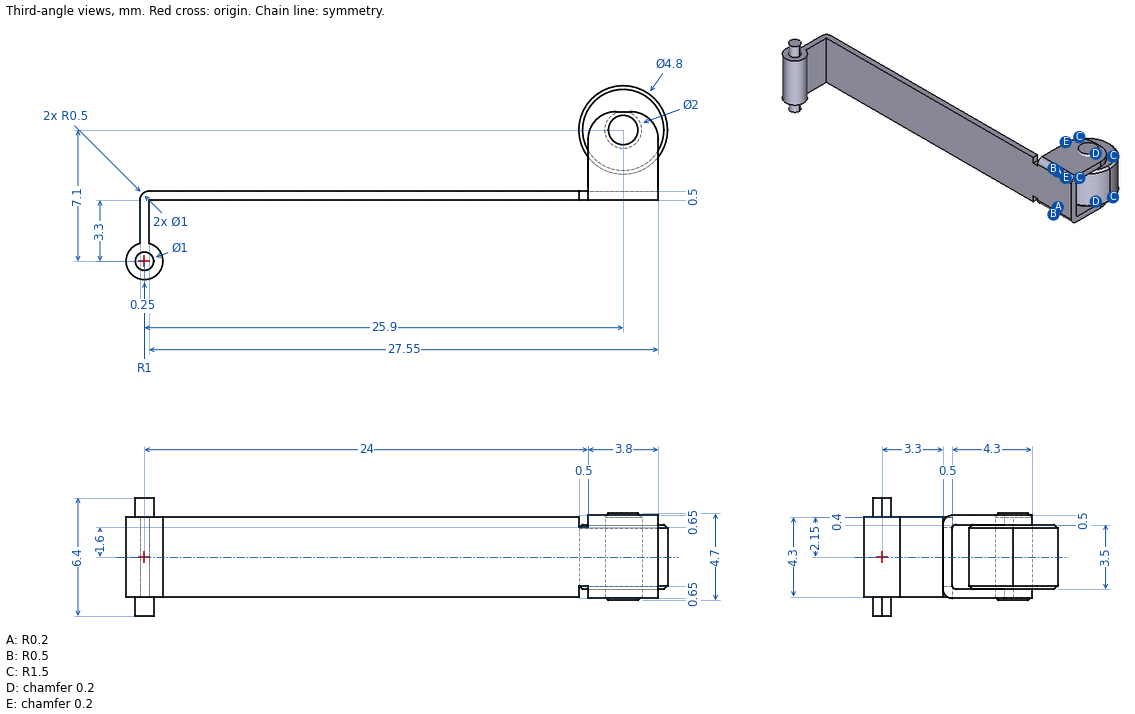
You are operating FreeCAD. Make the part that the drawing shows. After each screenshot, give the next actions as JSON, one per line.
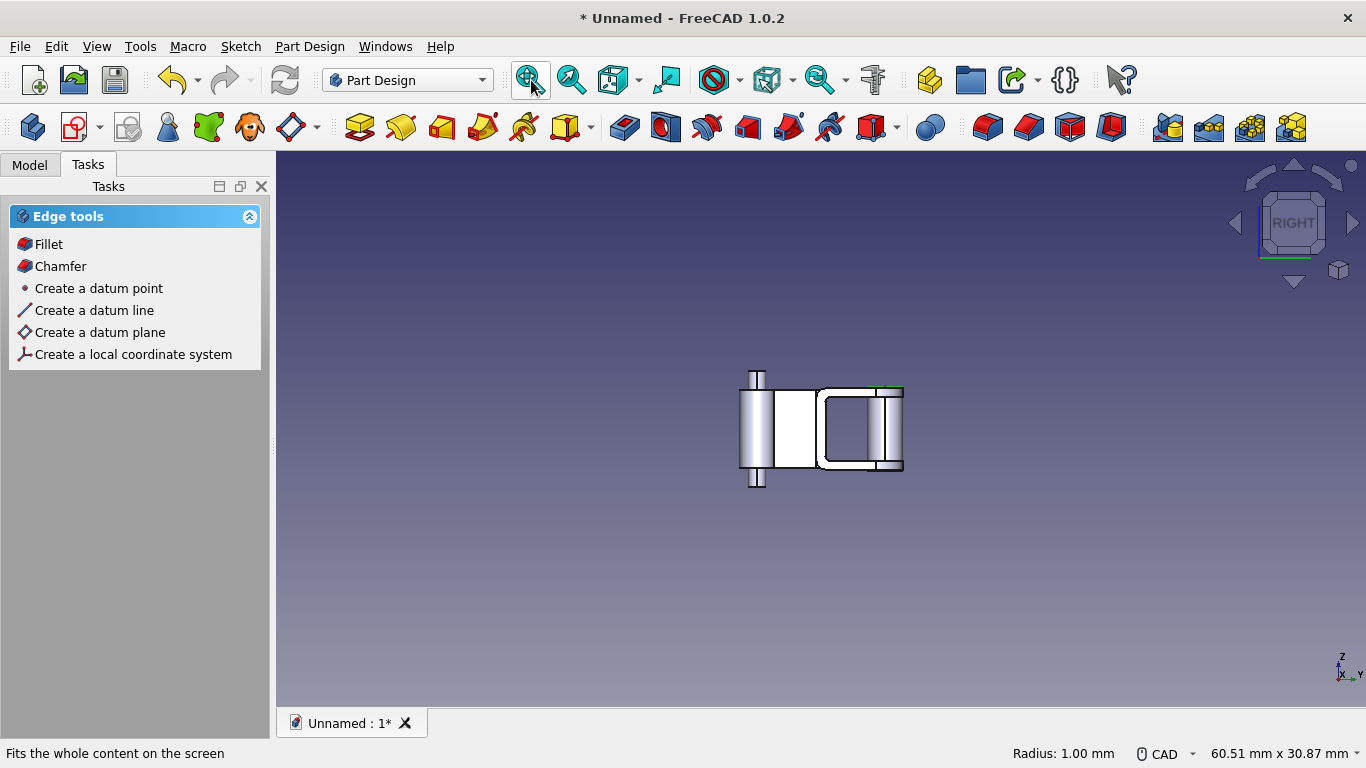
{"action": "key", "text": "5"}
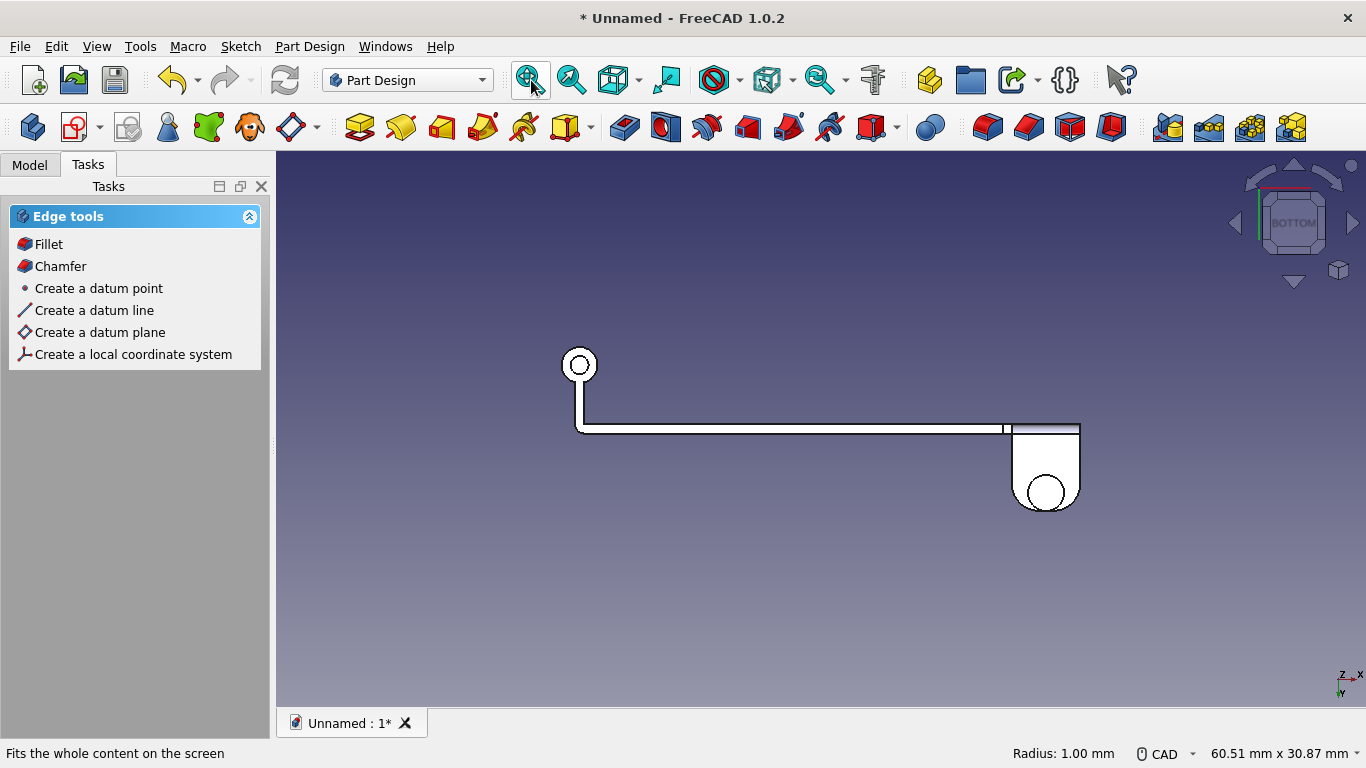
{"action": "left_click", "coordinate": [531, 80]}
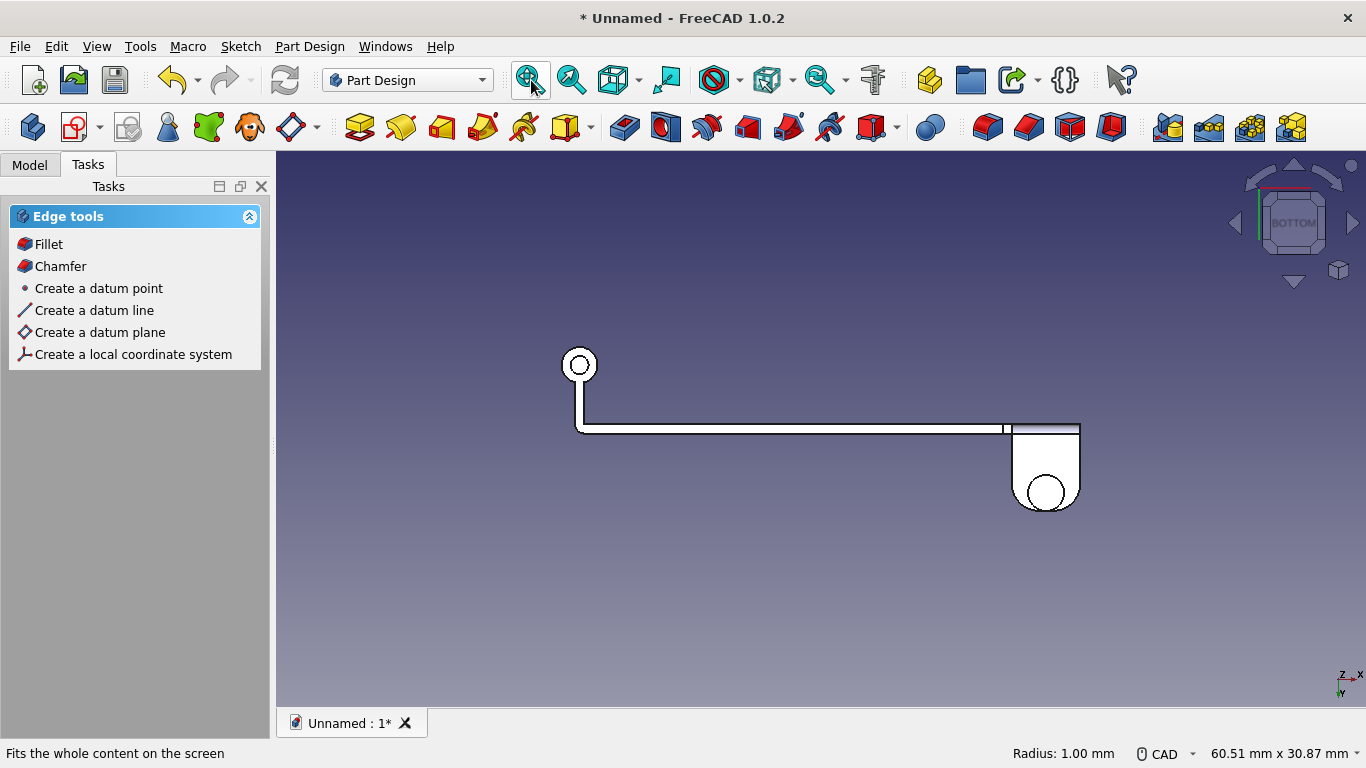
{"action": "left_click", "coordinate": [1028, 492], "text": "ctrl"}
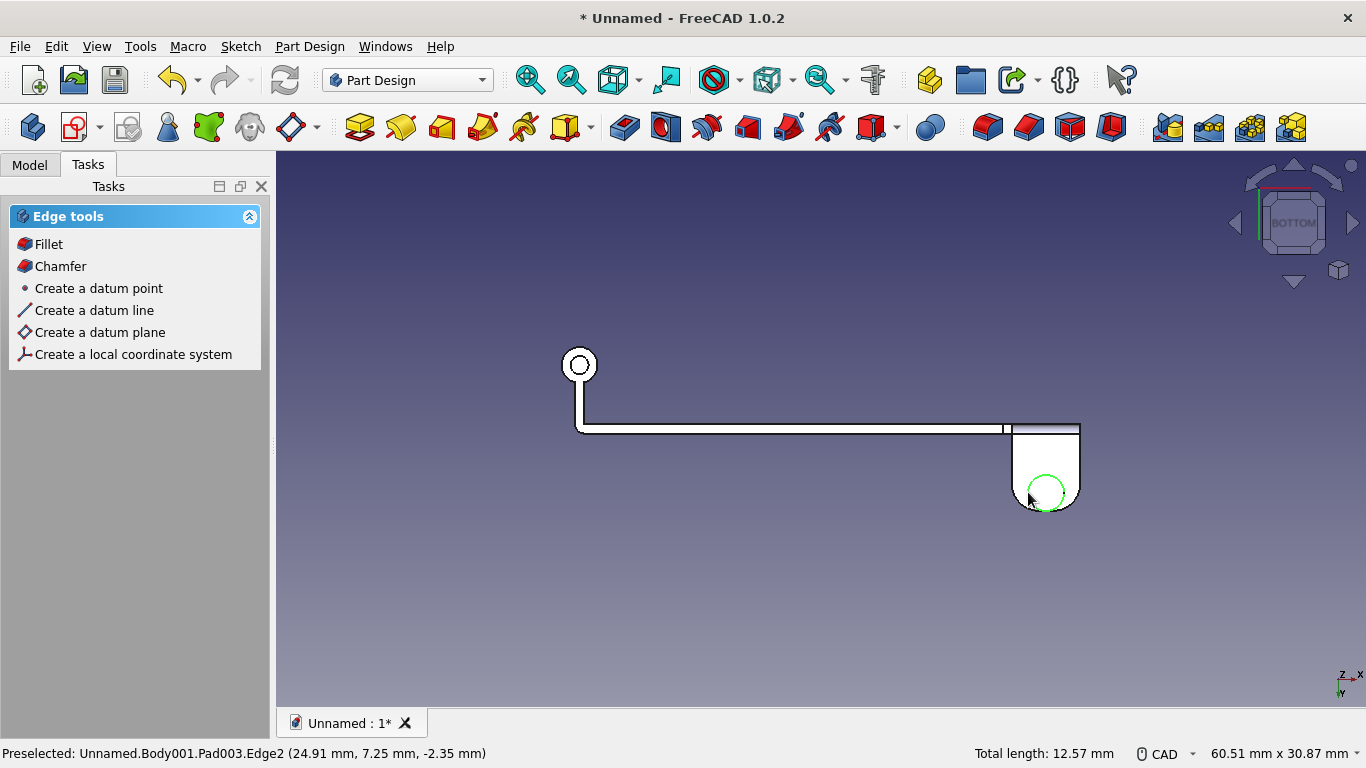
{"action": "left_click", "coordinate": [1029, 128]}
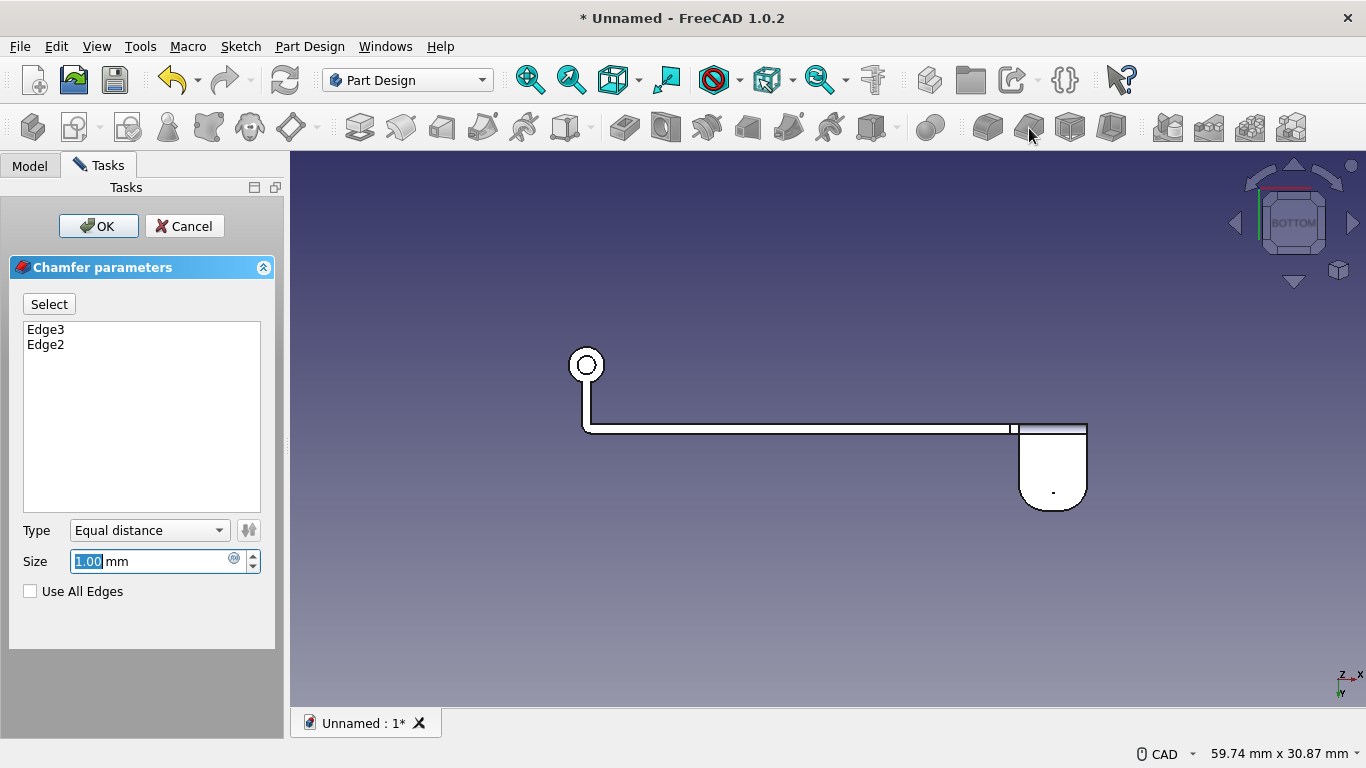
{"action": "type", "text": "0.2"}
{"action": "key", "text": "Tab"}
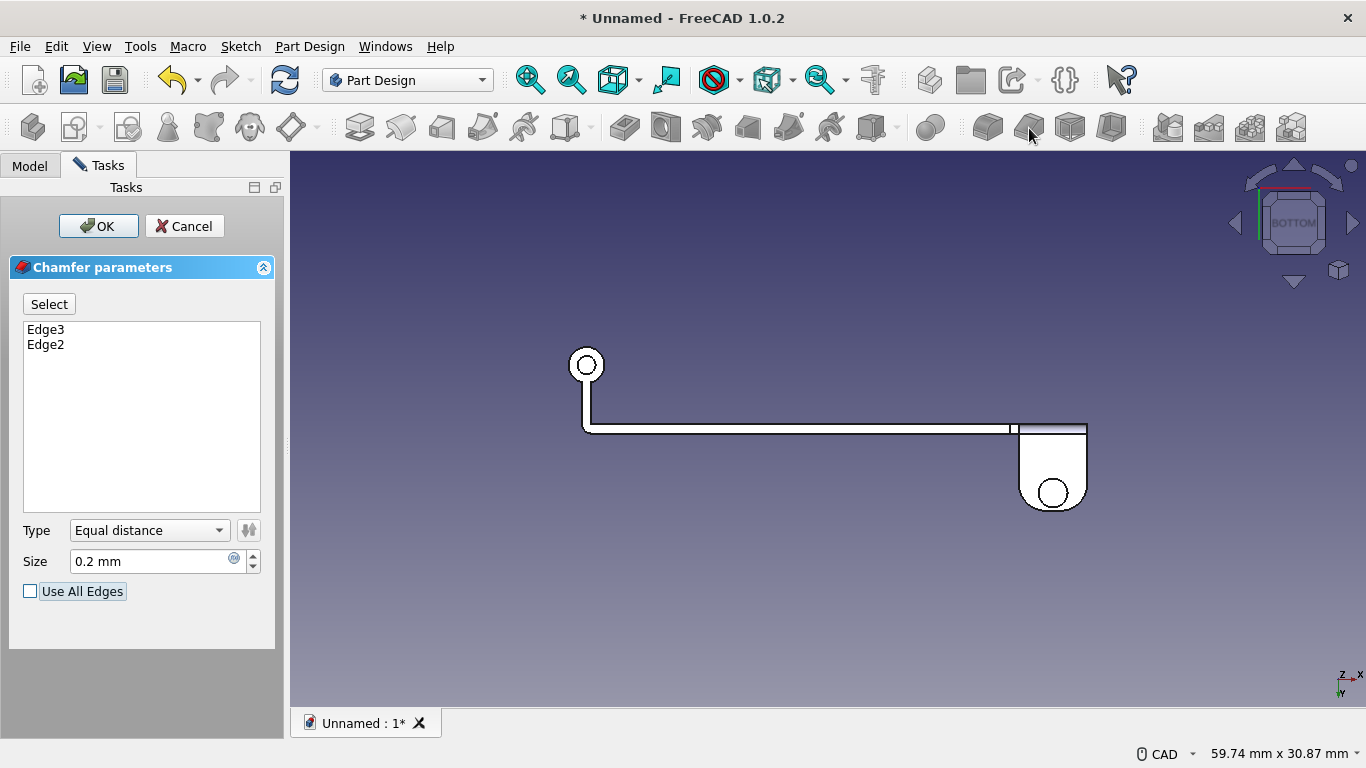
{"action": "left_click", "coordinate": [99, 226]}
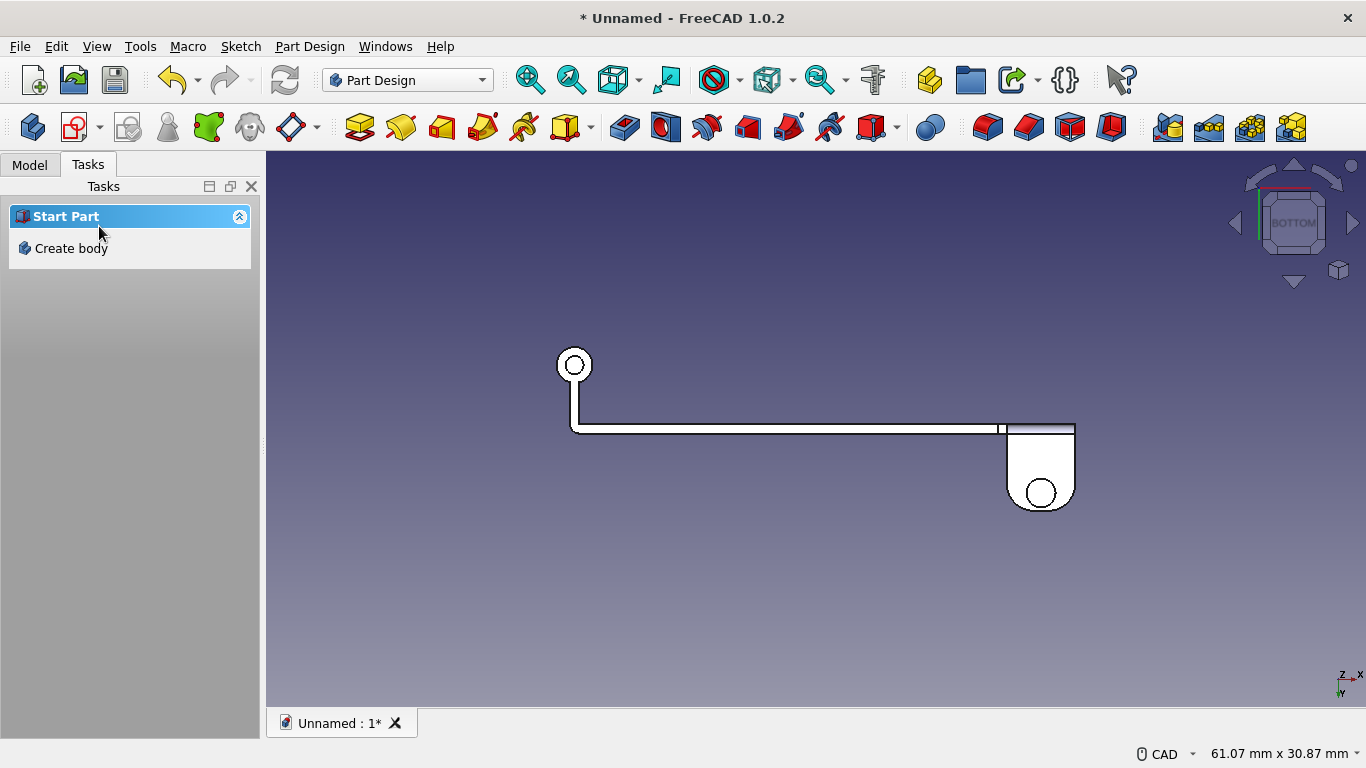
{"action": "key", "text": "v f"}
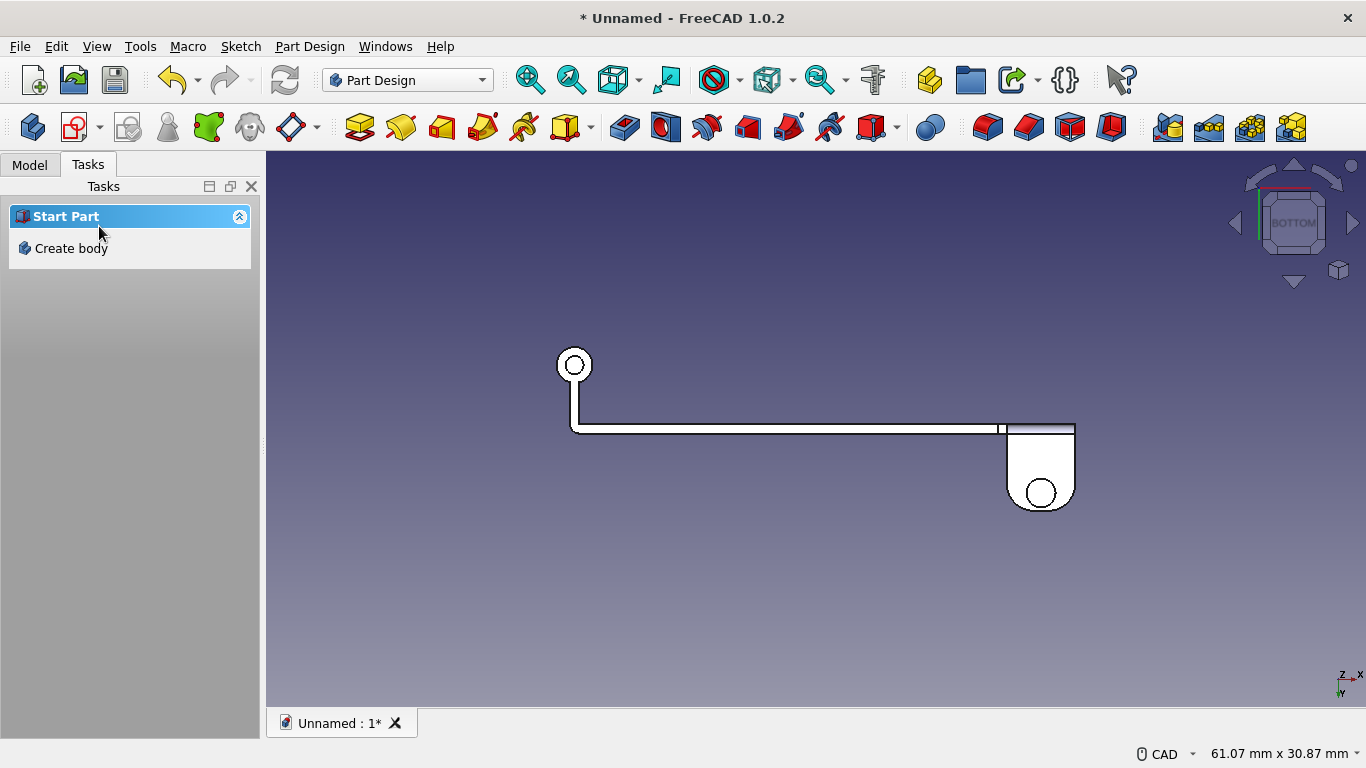
{"action": "left_click", "coordinate": [33, 128]}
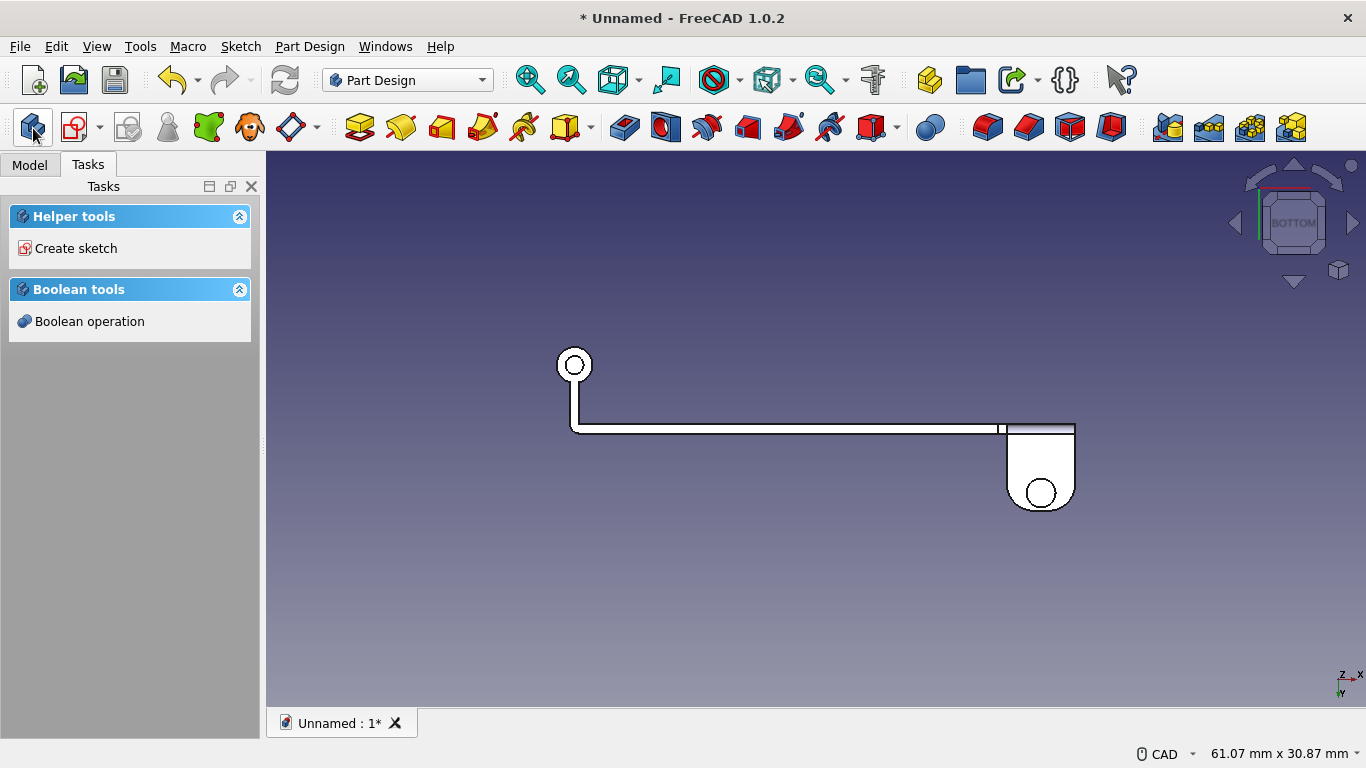
{"action": "left_click", "coordinate": [306, 667]}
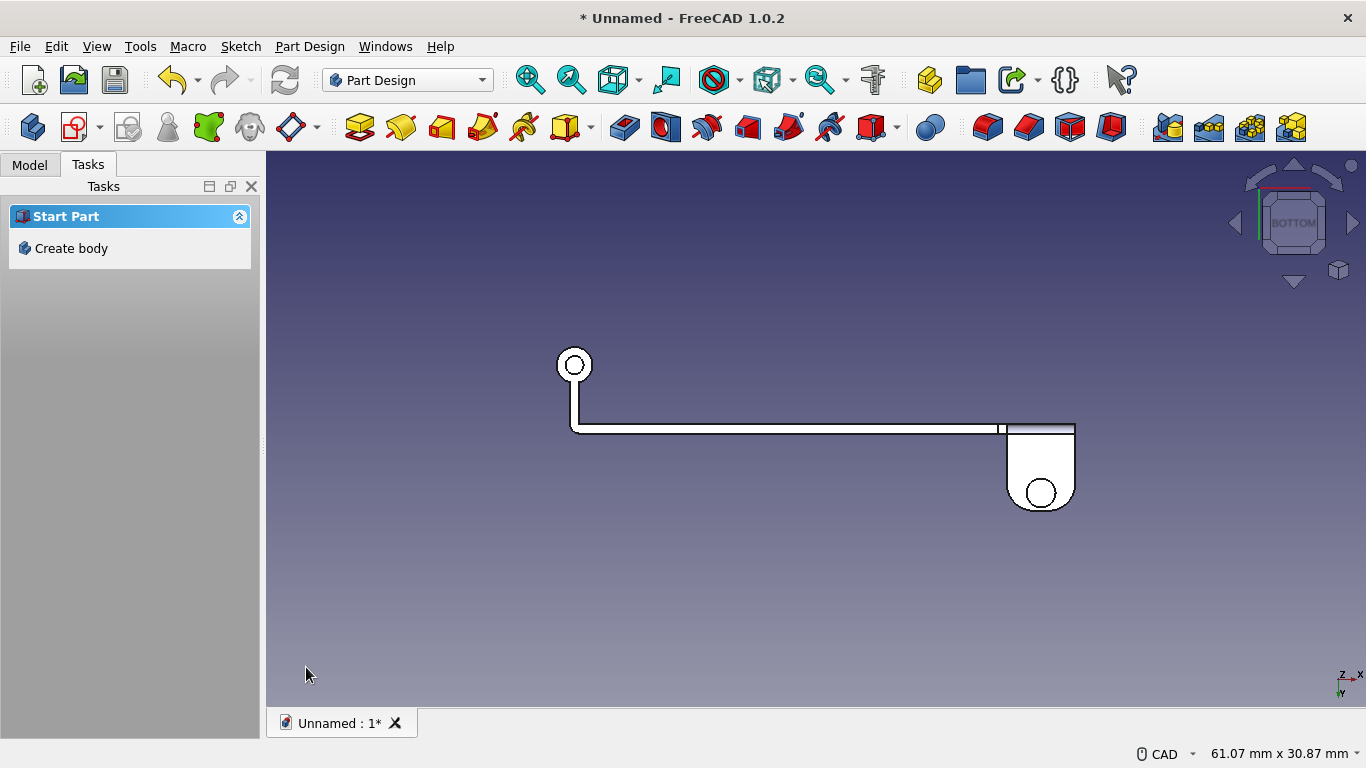
{"action": "left_click", "coordinate": [74, 128]}